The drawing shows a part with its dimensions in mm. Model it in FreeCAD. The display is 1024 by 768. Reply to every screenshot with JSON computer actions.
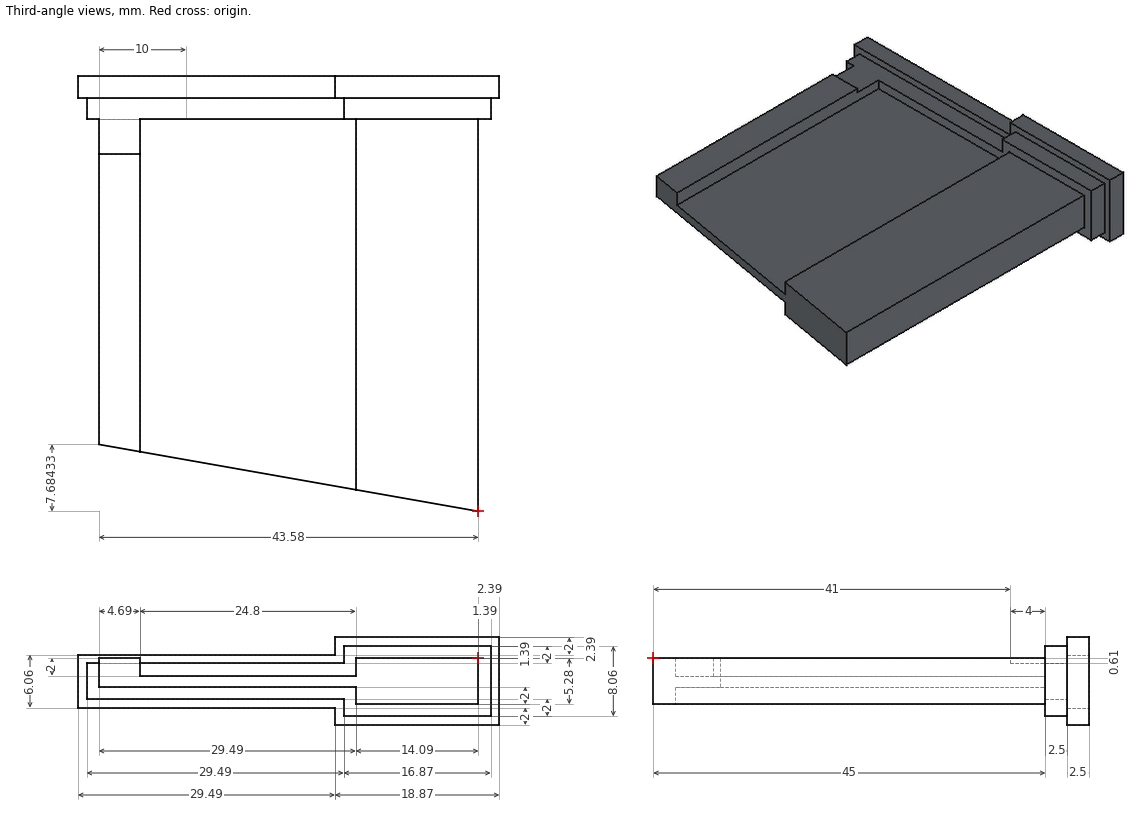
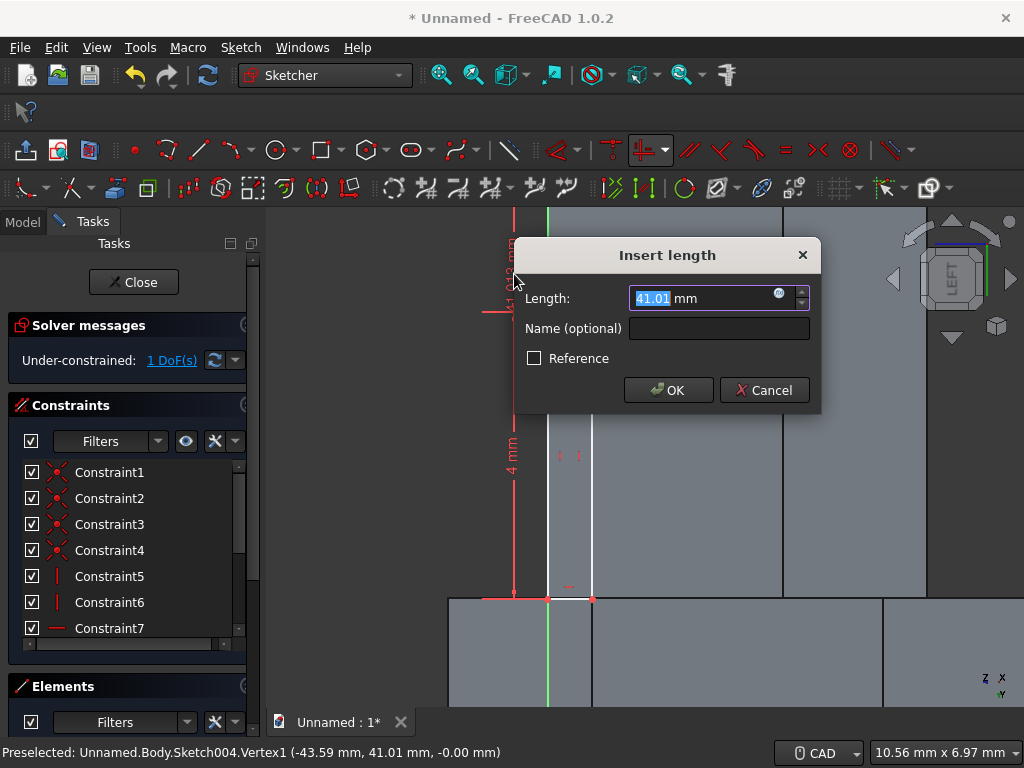
{"action": "type", "text": "41"}
{"action": "key", "text": "Return"}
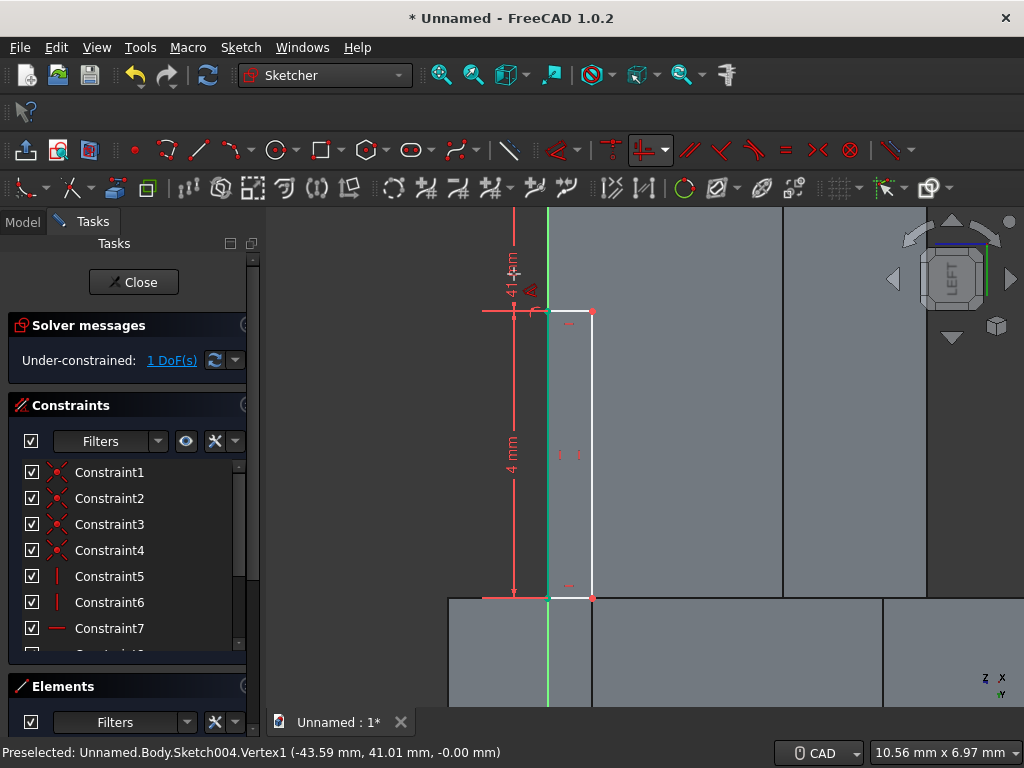
{"action": "left_click", "coordinate": [561, 598]}
{"action": "left_click", "coordinate": [570, 632]}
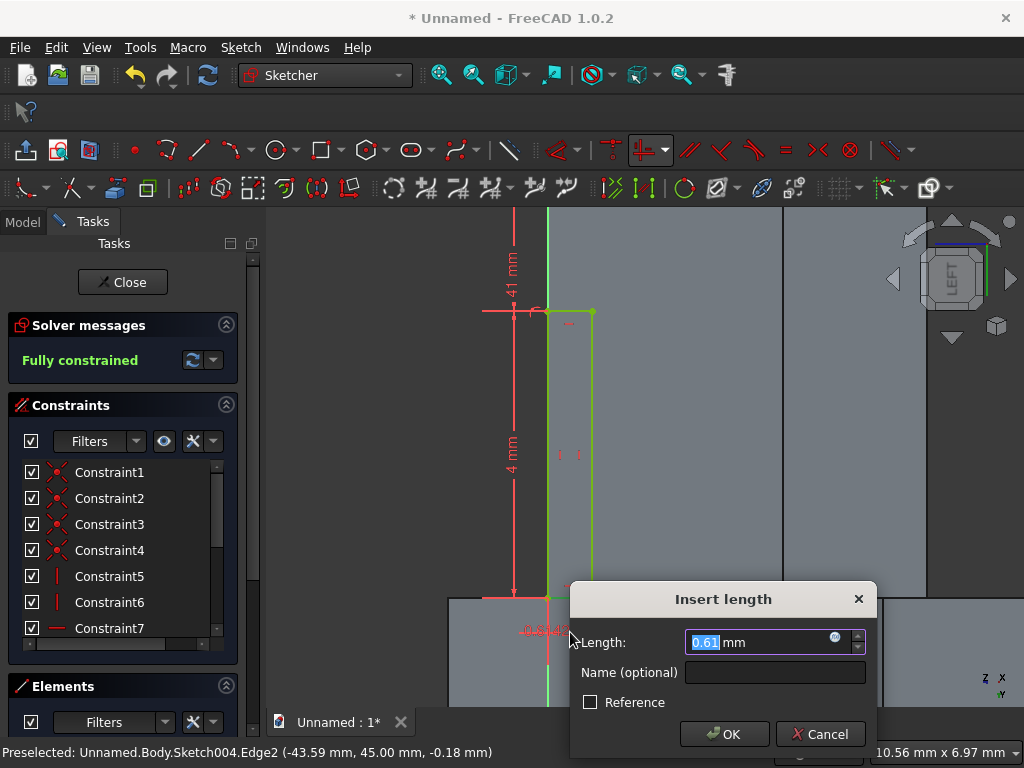
{"action": "type", "text": "0.61"}
{"action": "key", "text": "Return"}
{"action": "key", "text": "Escape"}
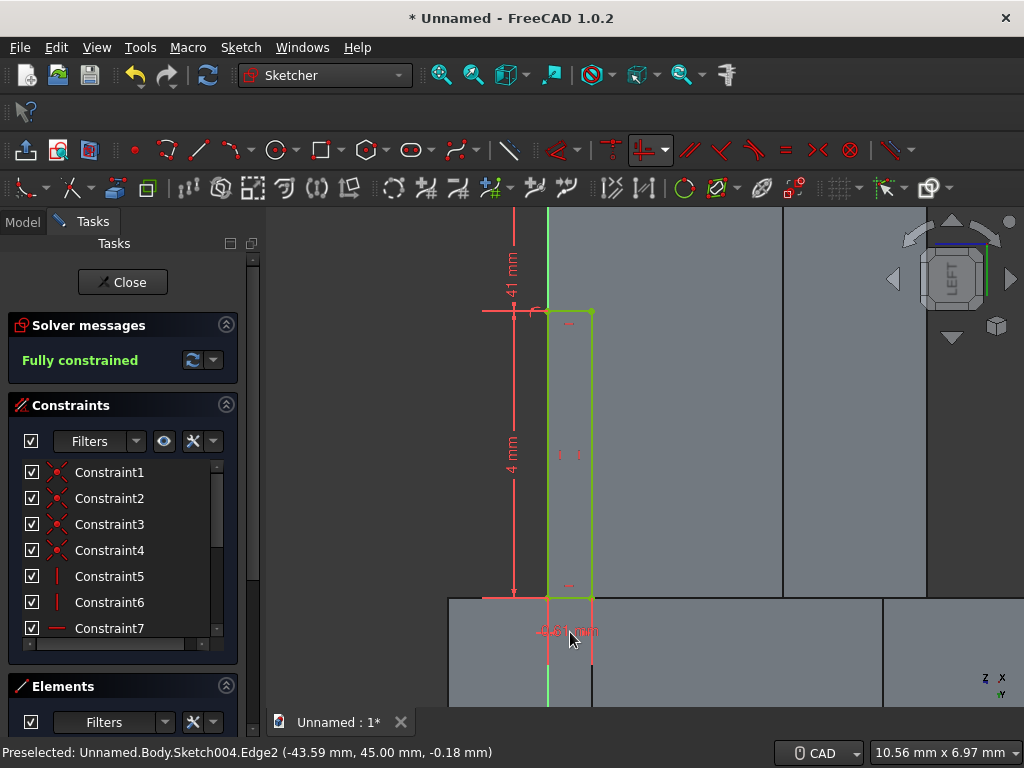
{"action": "left_click", "coordinate": [123, 282]}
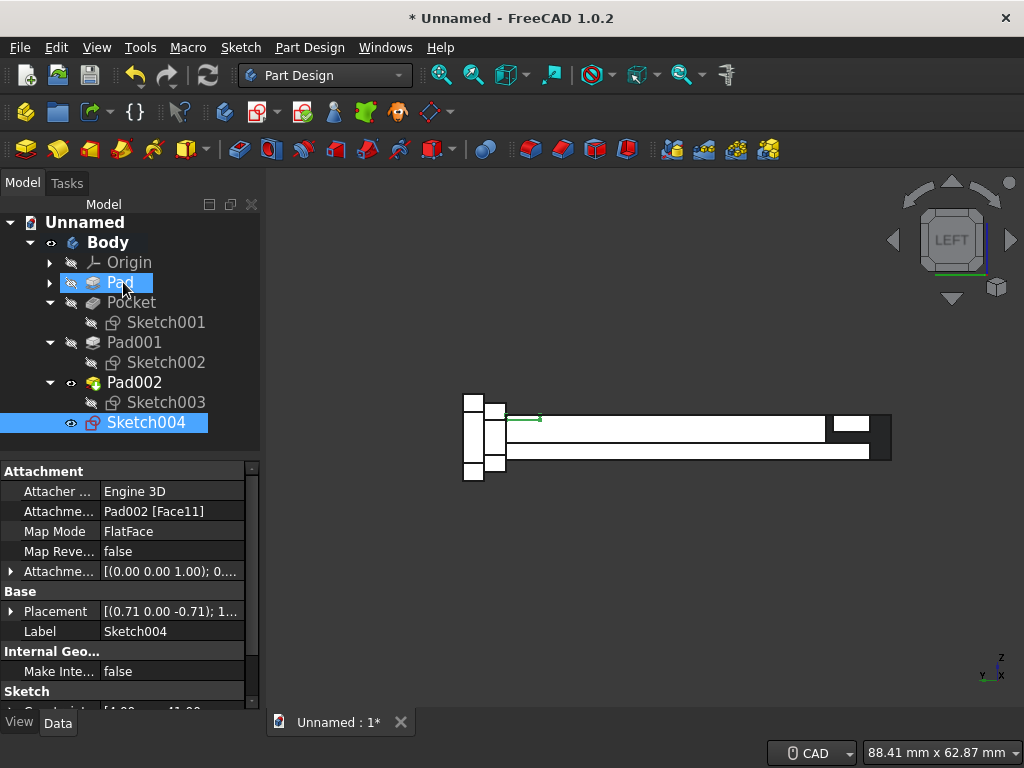
{"action": "left_click", "coordinate": [240, 150]}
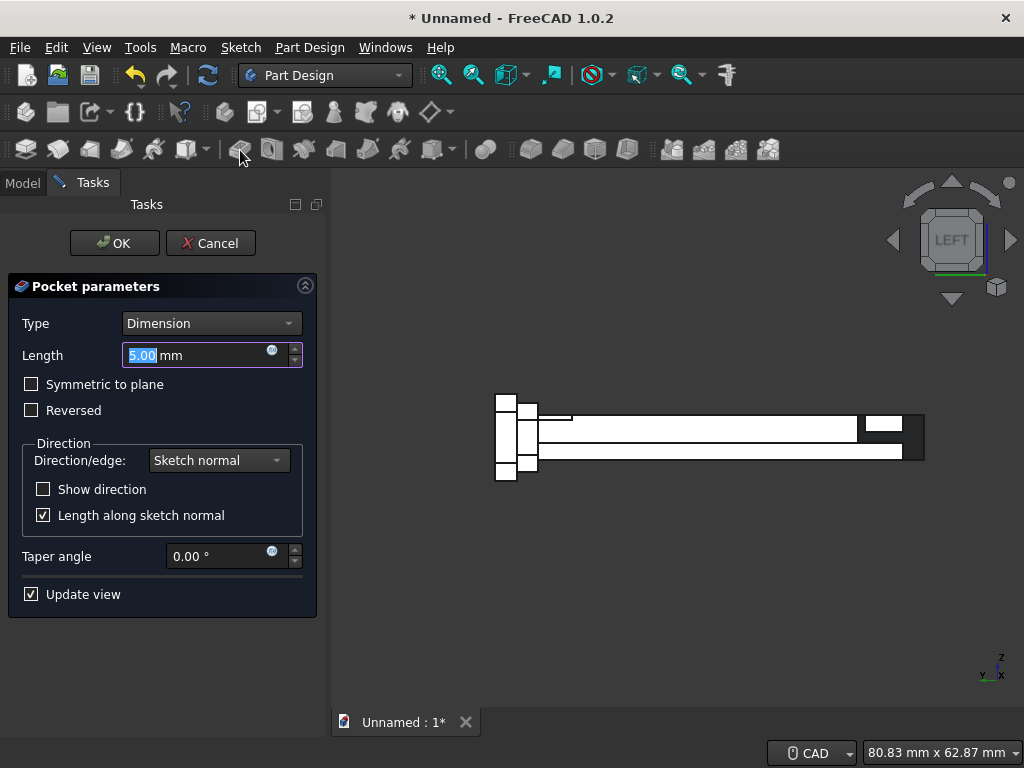
{"action": "type", "text": "10"}
{"action": "key", "text": "Tab"}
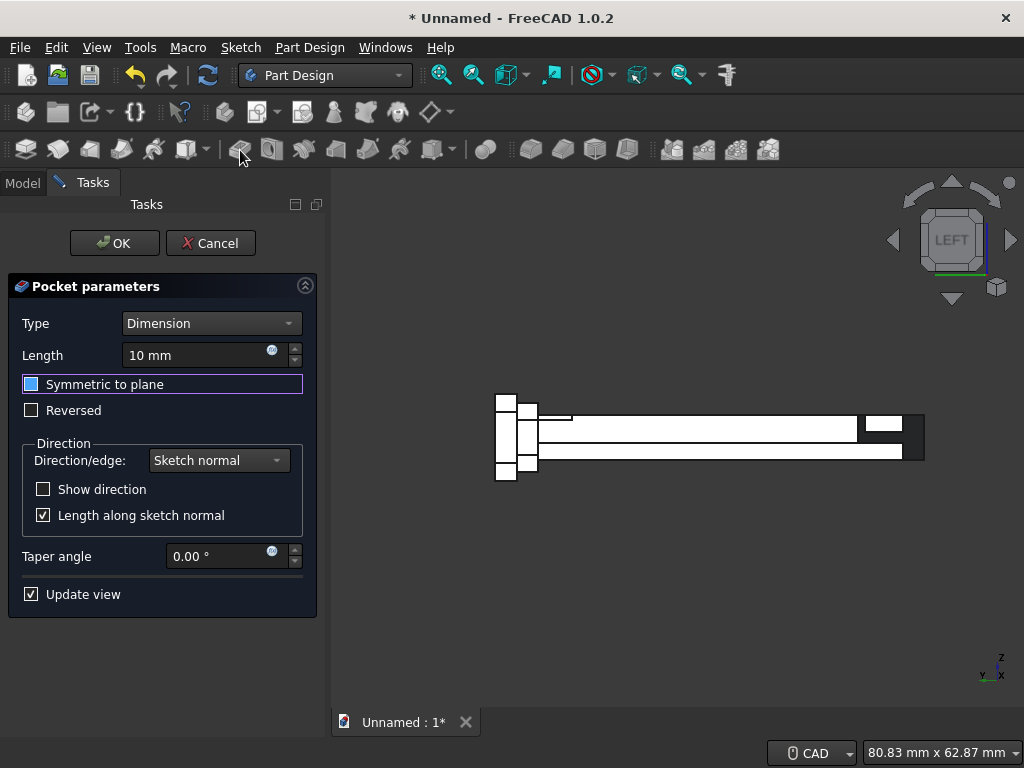
{"action": "left_click", "coordinate": [115, 243]}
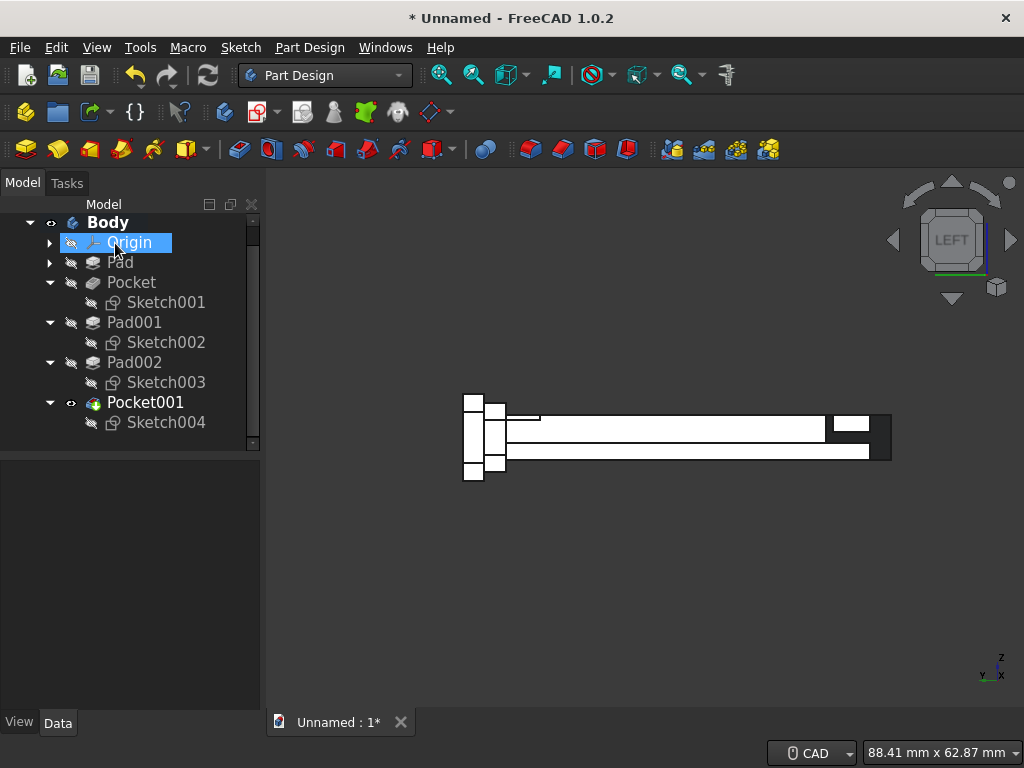
{"action": "key", "text": "0"}